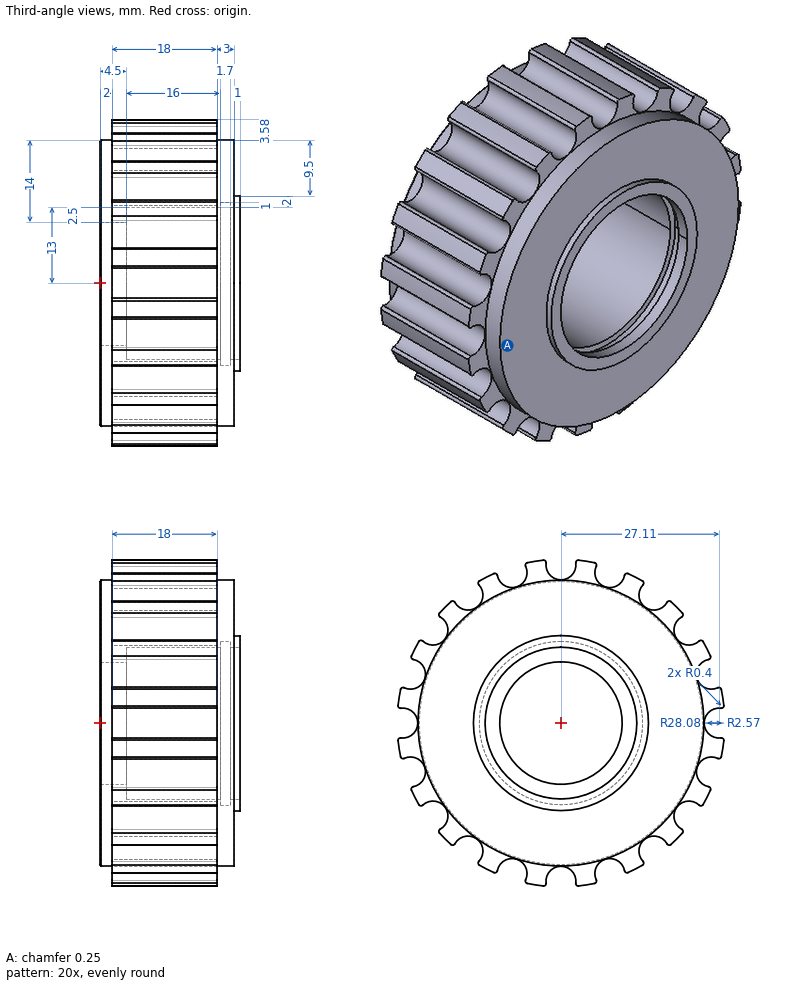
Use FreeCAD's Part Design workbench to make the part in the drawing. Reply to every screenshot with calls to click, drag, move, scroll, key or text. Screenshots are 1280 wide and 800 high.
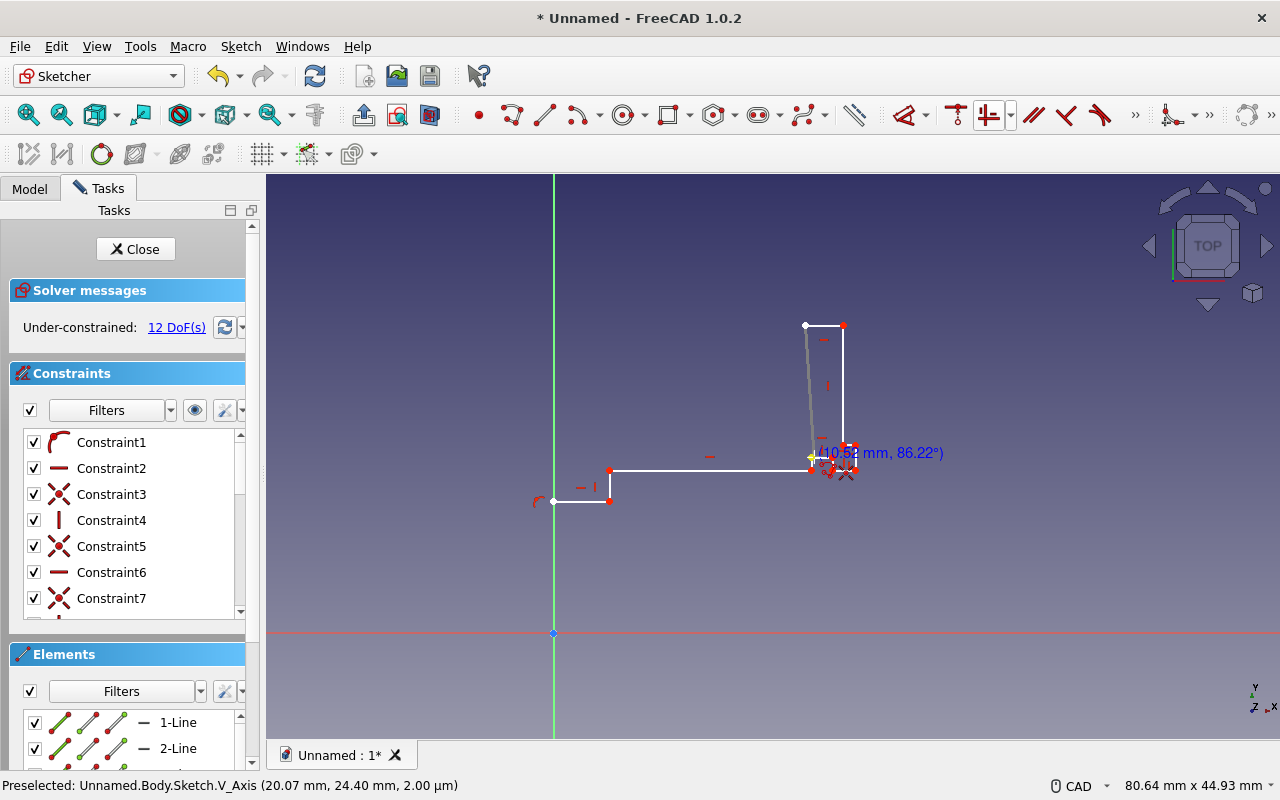
click(805, 280)
click(579, 280)
click(579, 325)
click(563, 325)
click(554, 502)
key(Escape)
key(Escape)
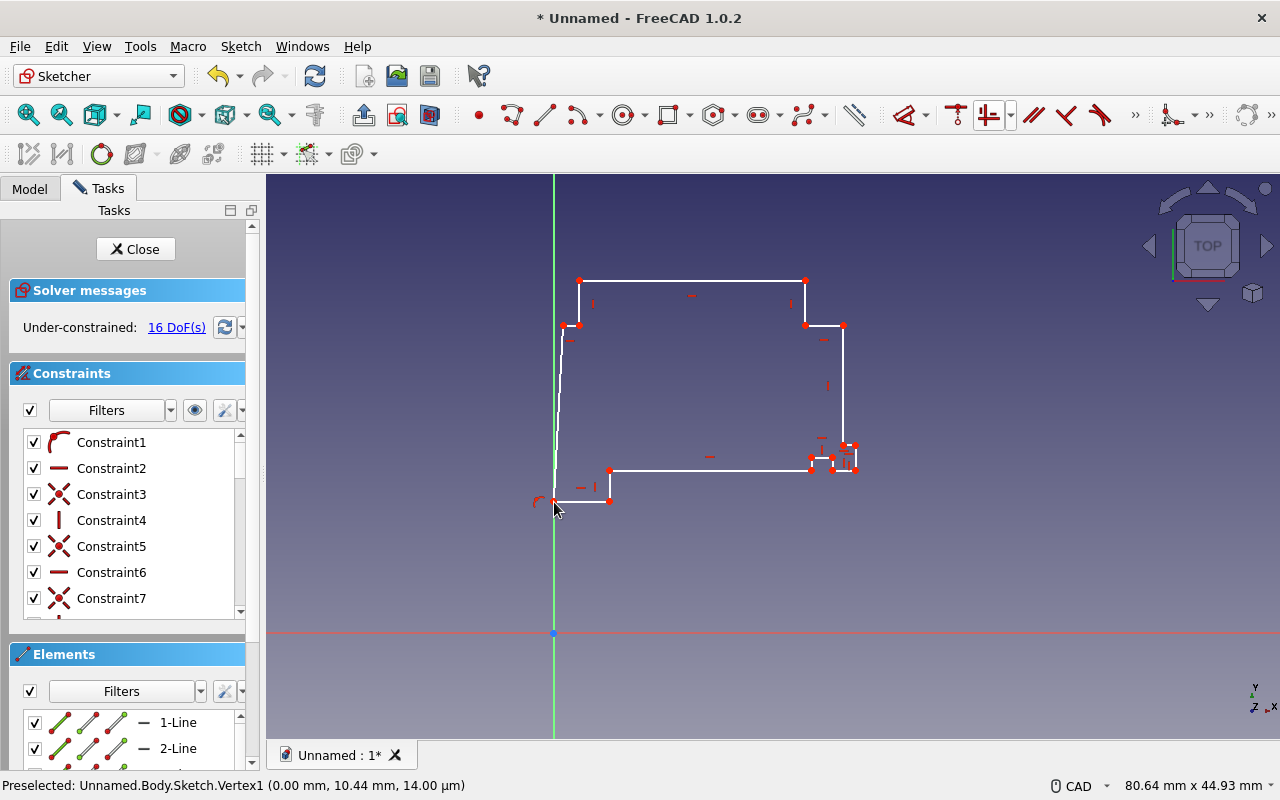
click(557, 449)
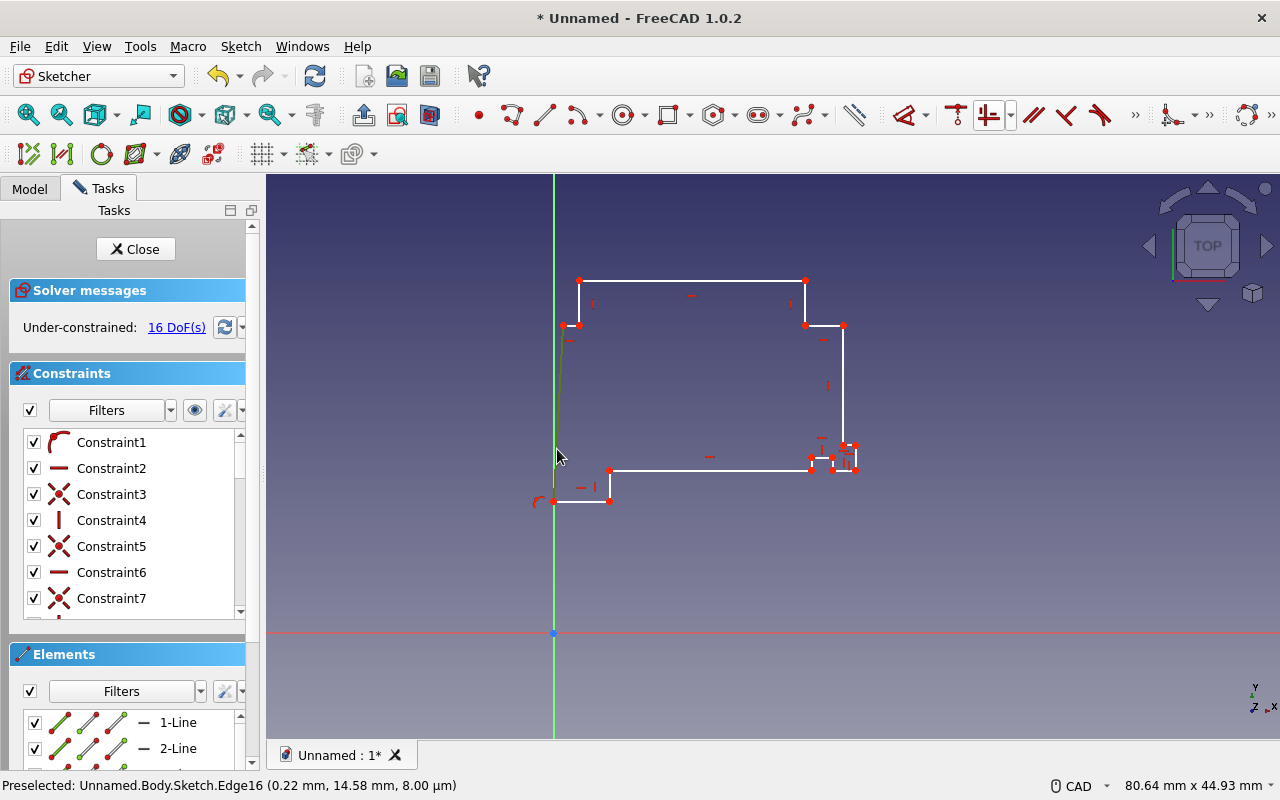
key(v)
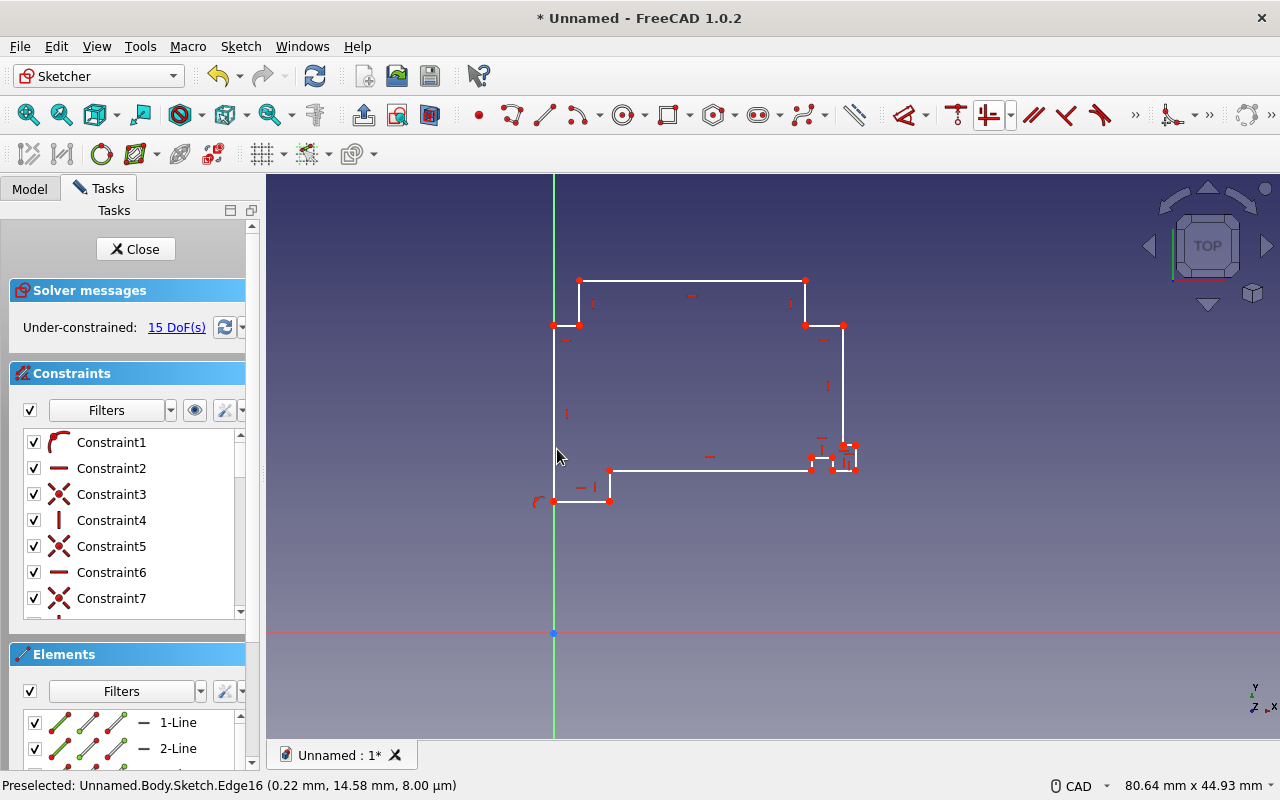
click(904, 116)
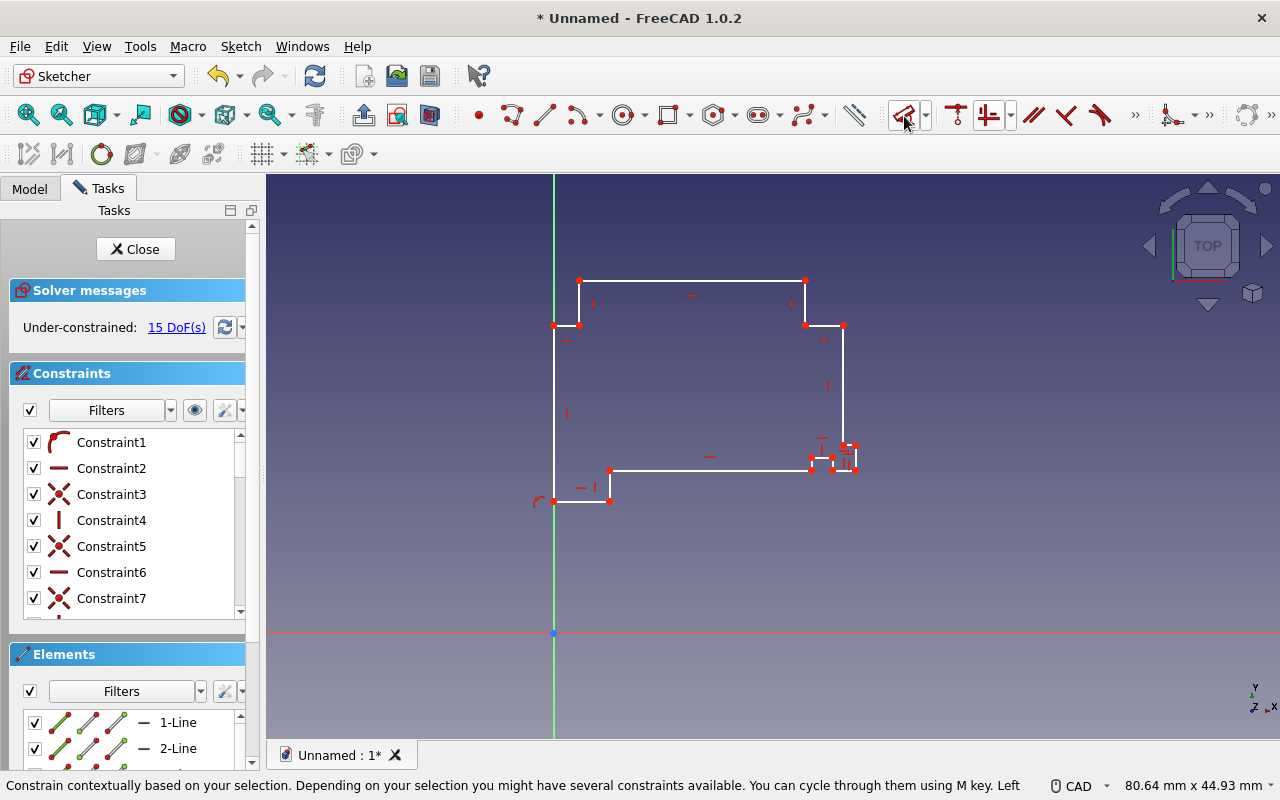
scroll(812, 464, up, 6)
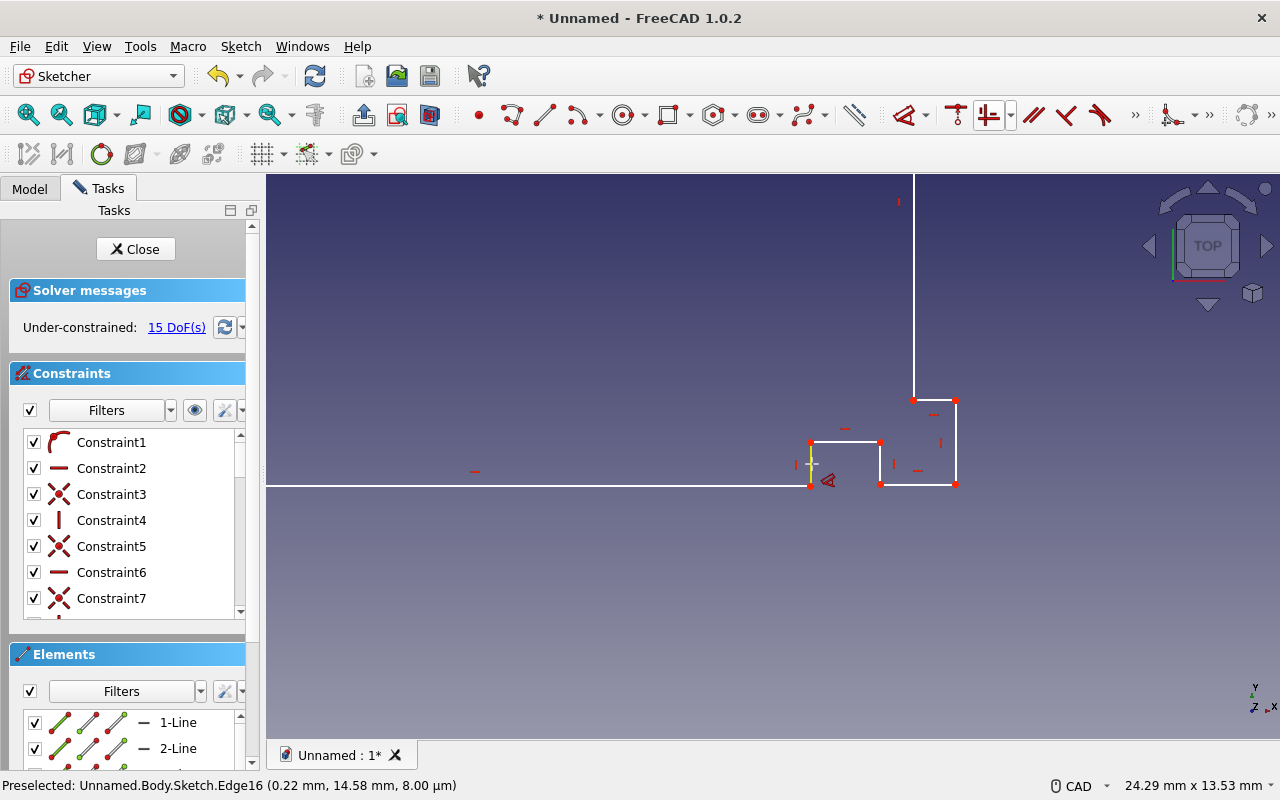
click(811, 464)
click(845, 464)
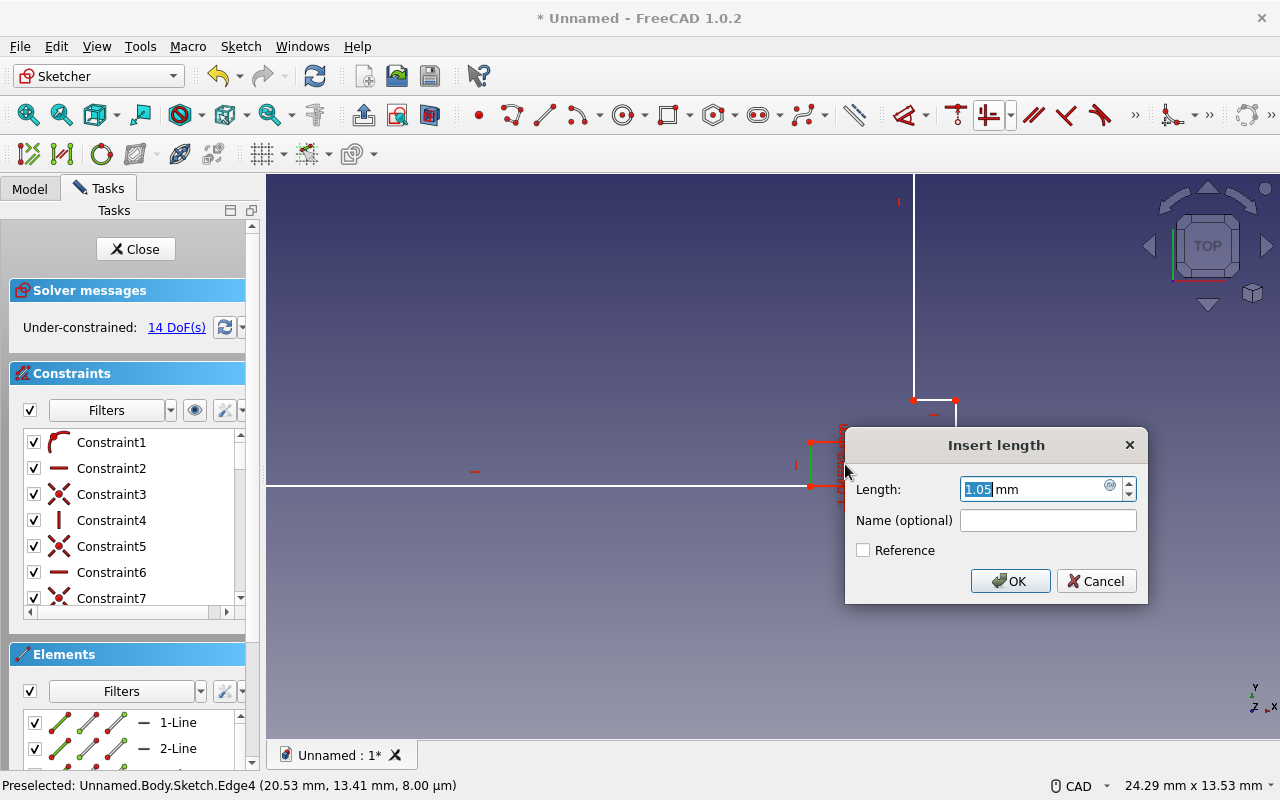
text(1)
key(Return)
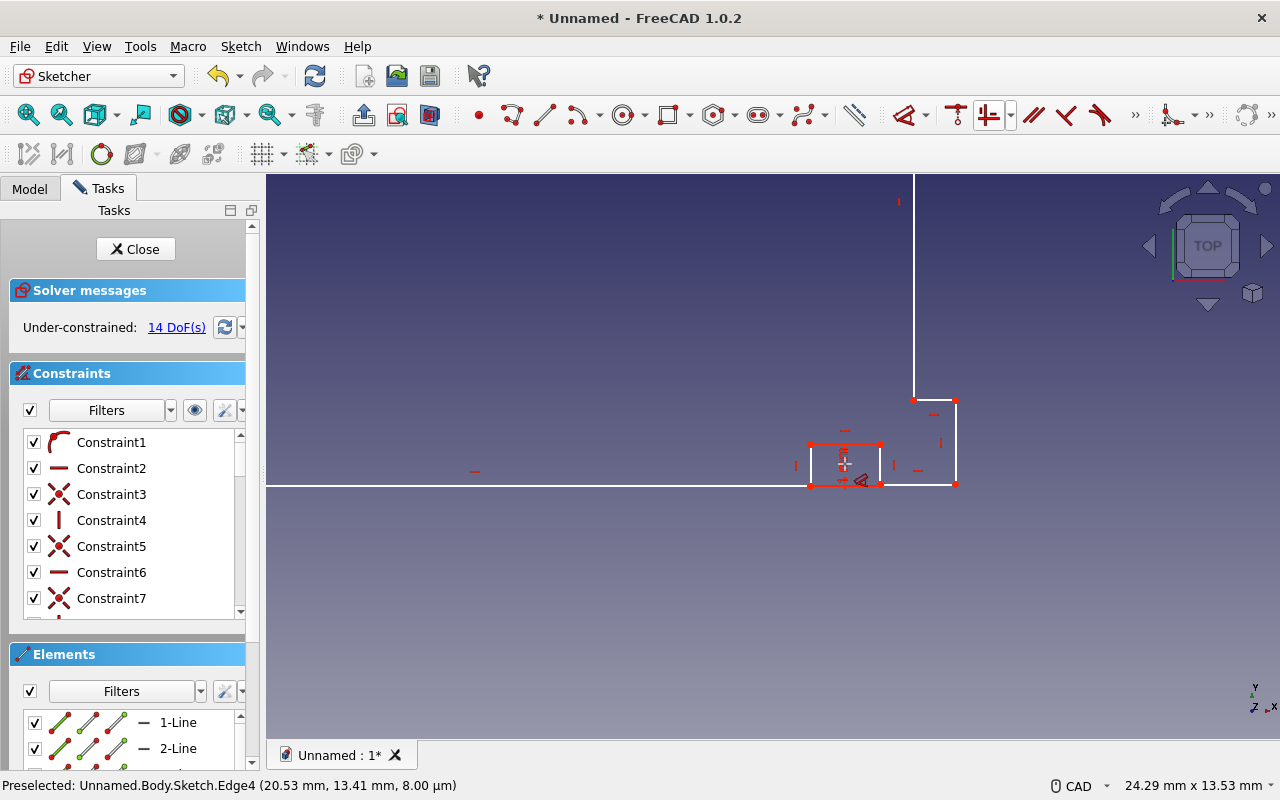
click(880, 456)
click(938, 464)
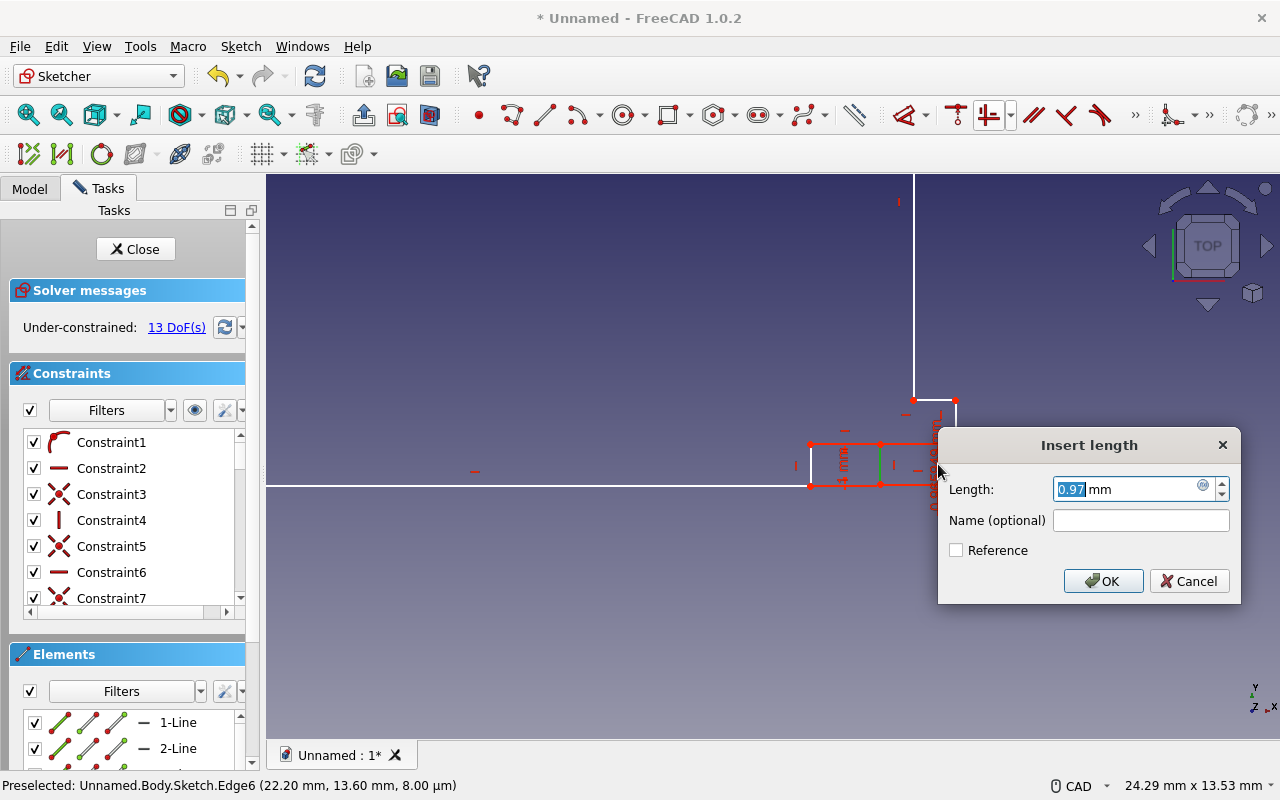
text(1)
key(Return)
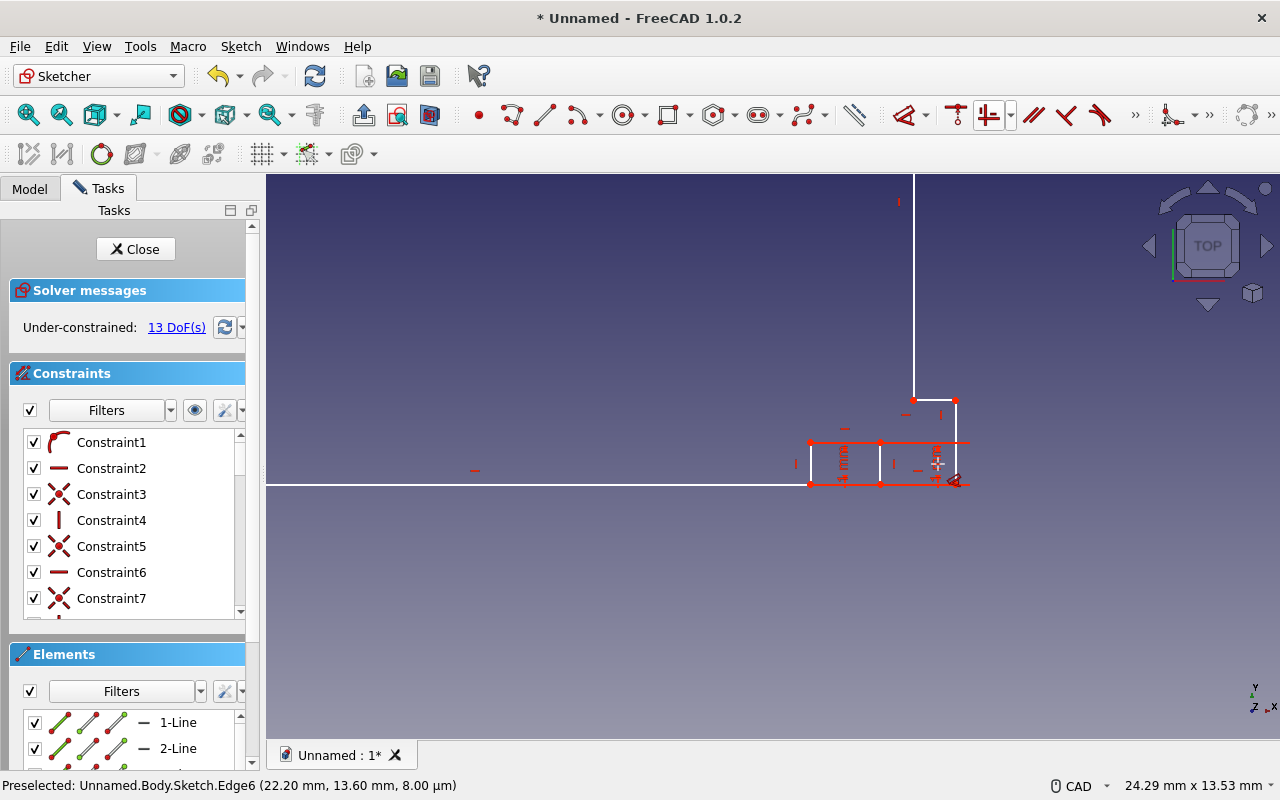
click(956, 459)
click(990, 442)